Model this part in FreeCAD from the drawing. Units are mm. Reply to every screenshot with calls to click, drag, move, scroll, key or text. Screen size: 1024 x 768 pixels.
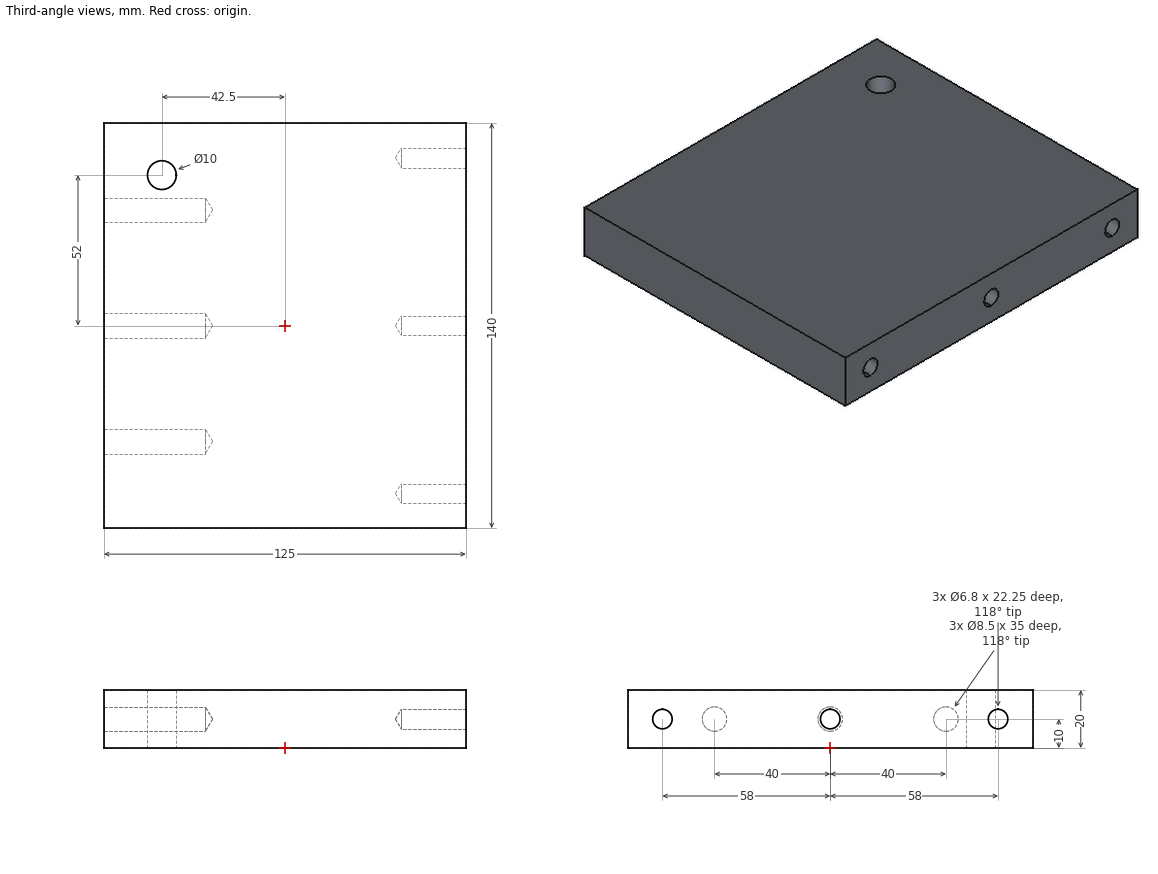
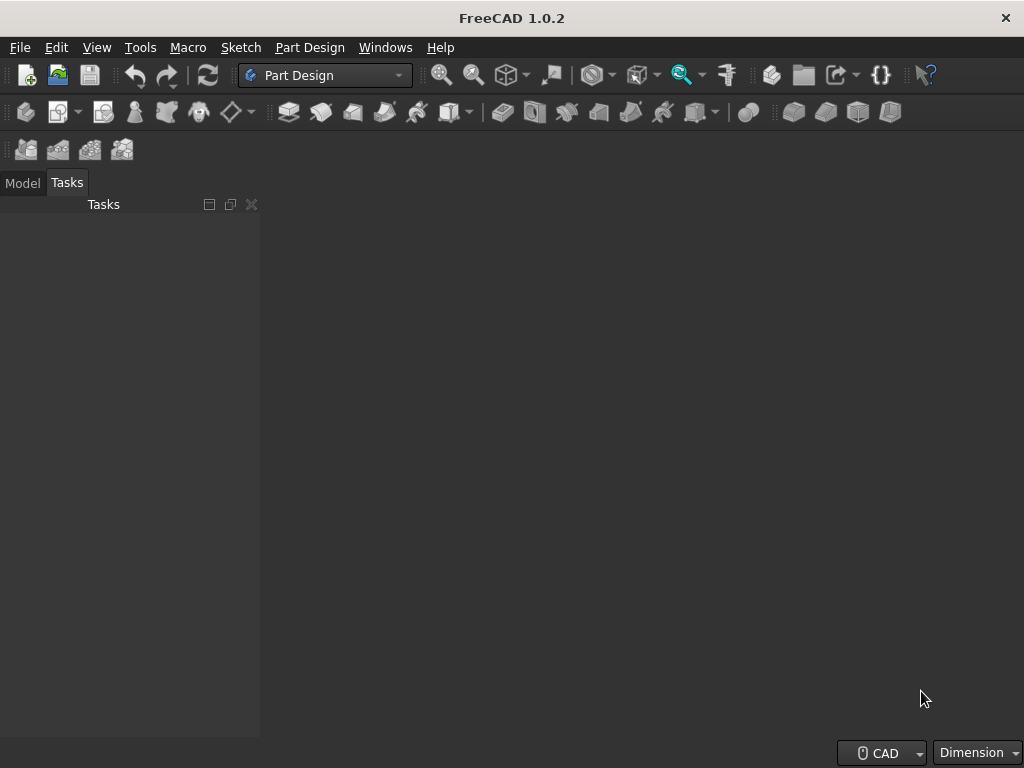
click(26, 76)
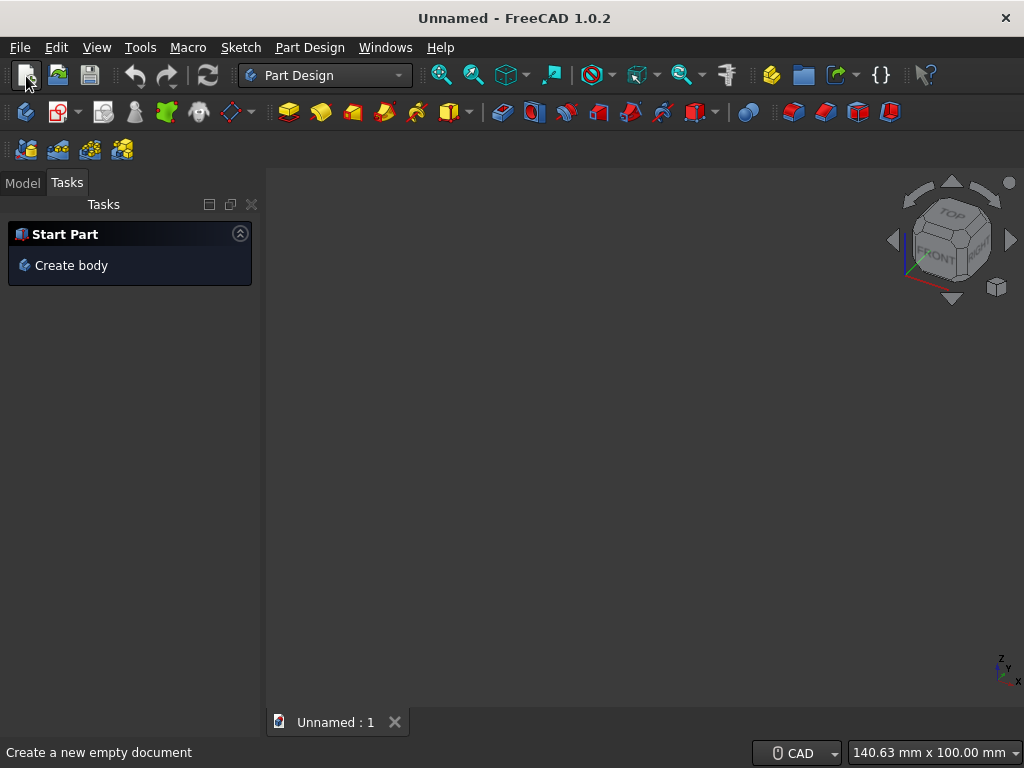
click(58, 112)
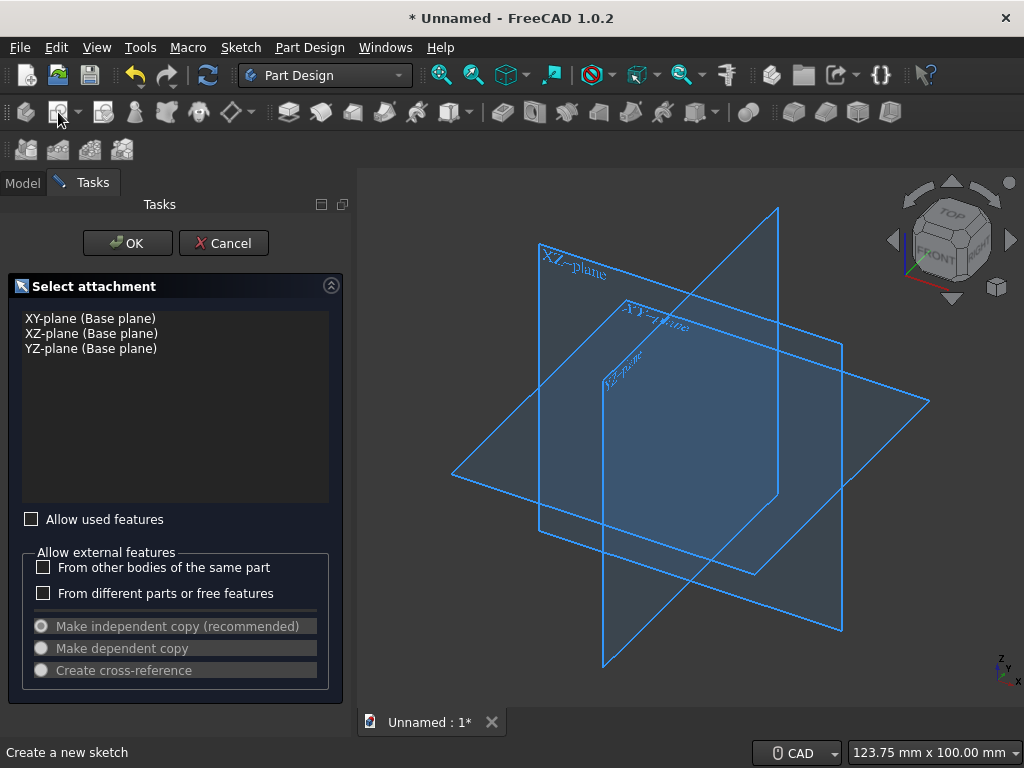
click(82, 318)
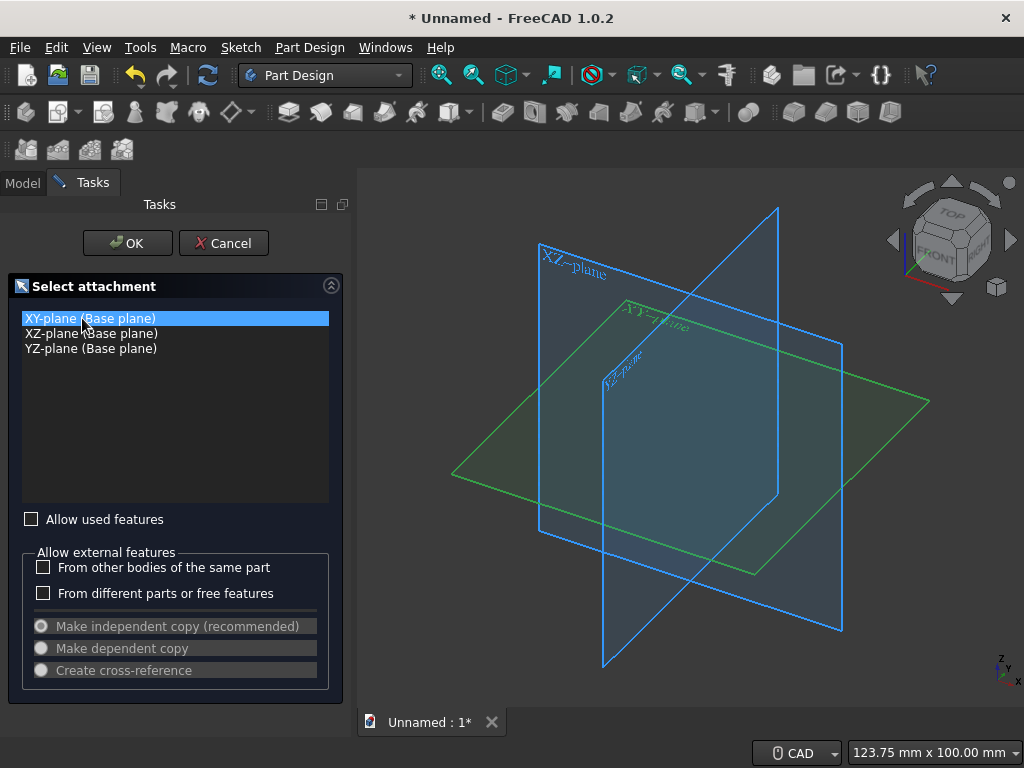
click(128, 243)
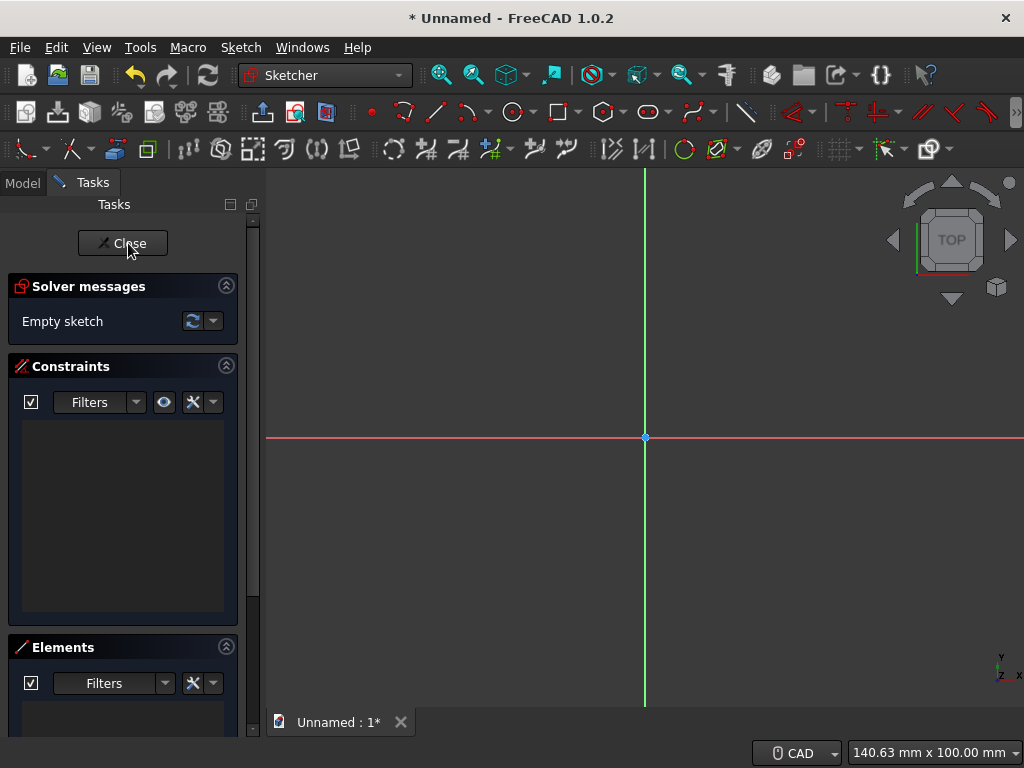
scroll(521, 438, down, 4)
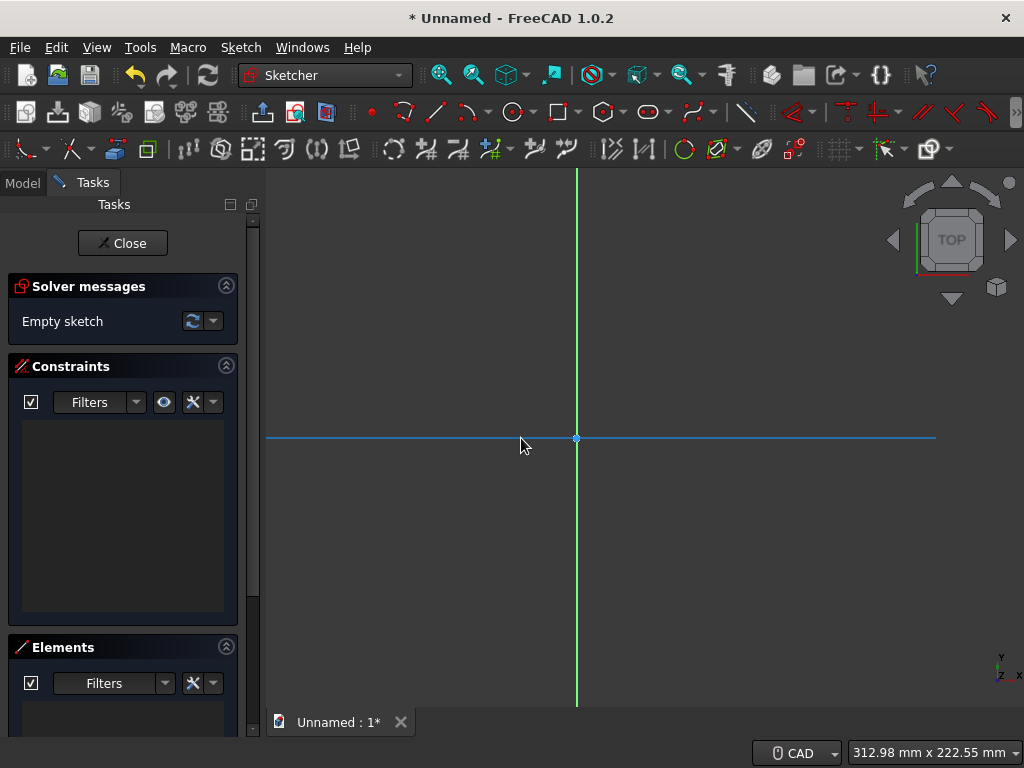
click(580, 112)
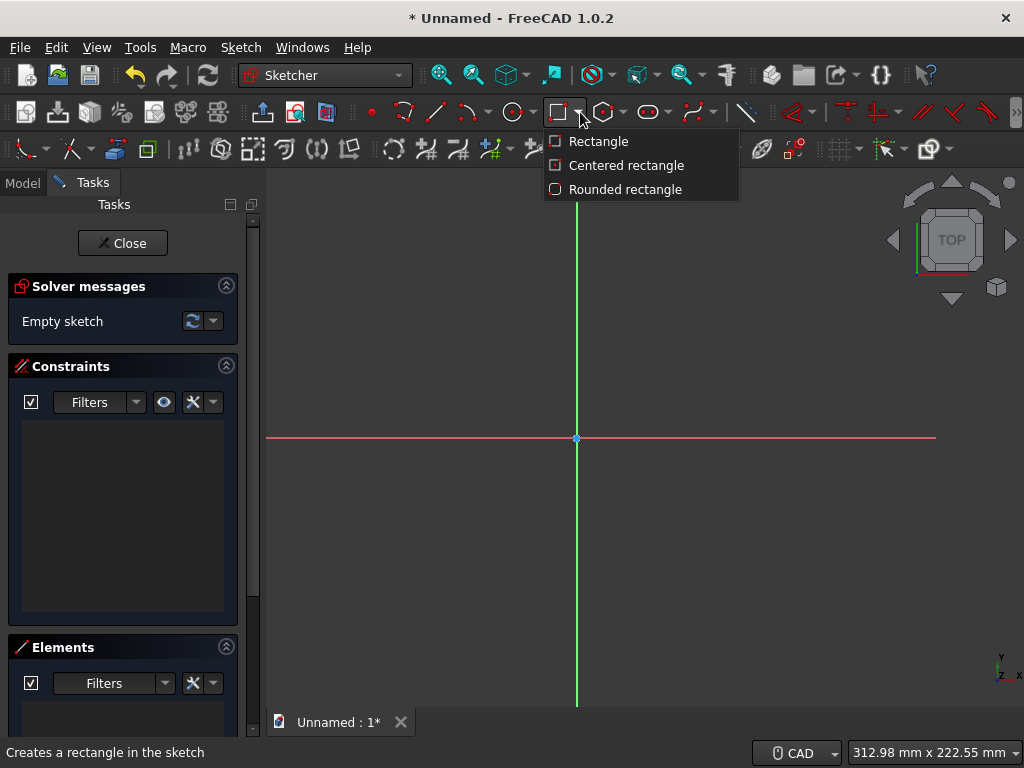
click(642, 165)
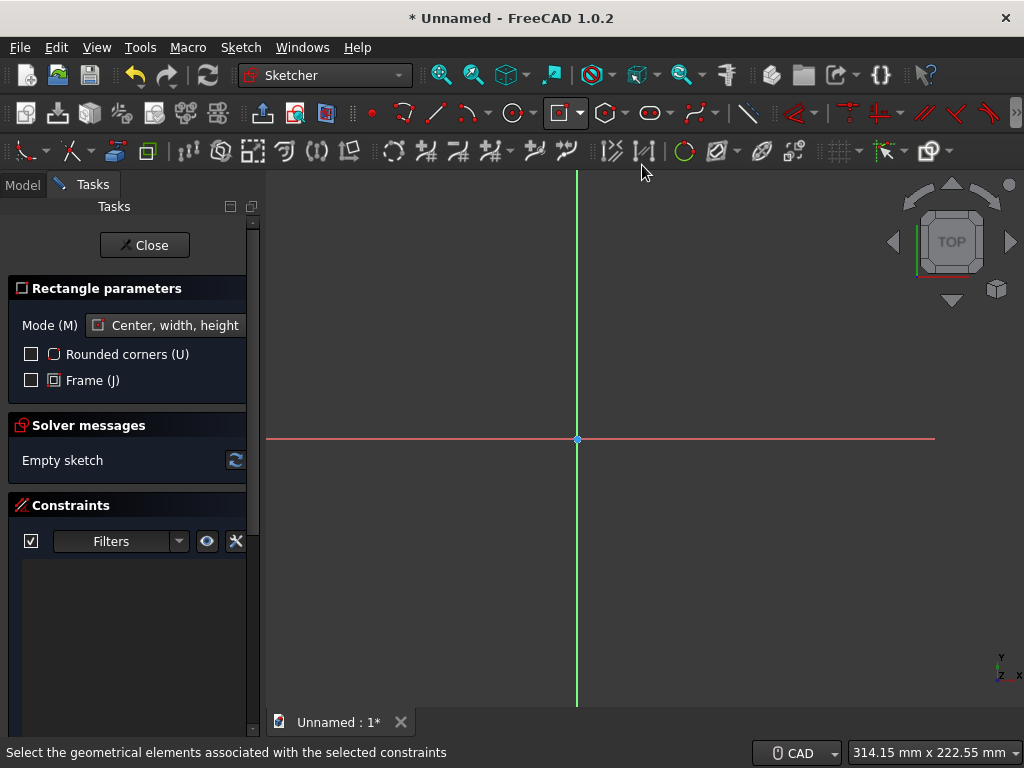
click(577, 439)
click(728, 270)
key(Escape)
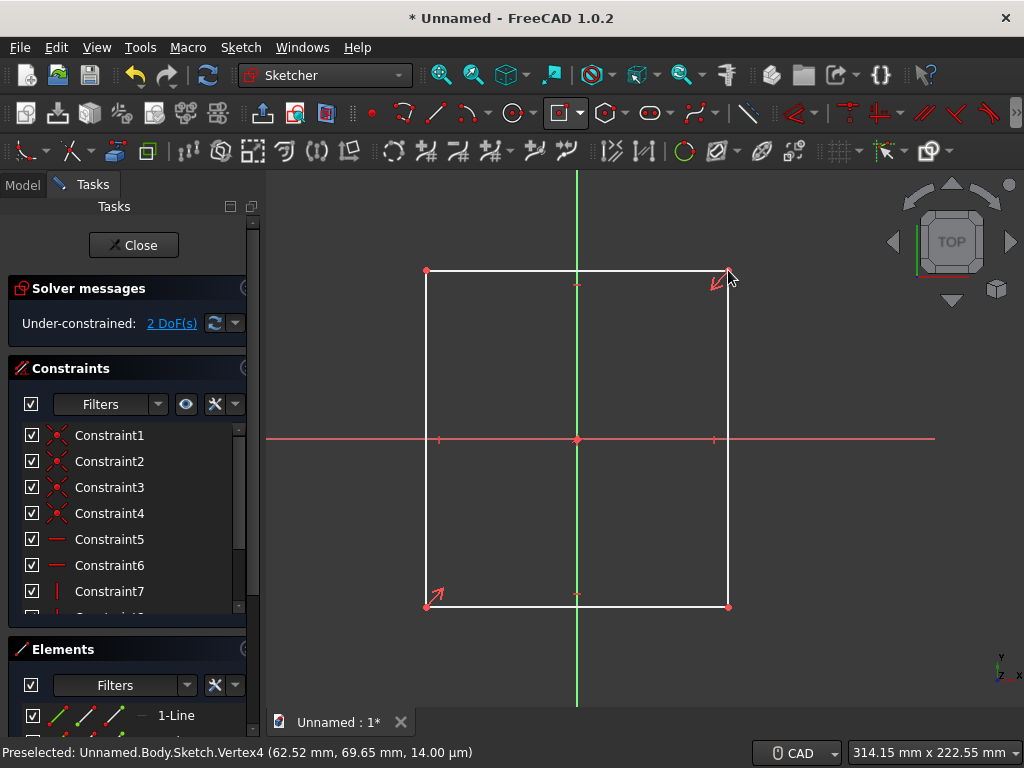
click(794, 114)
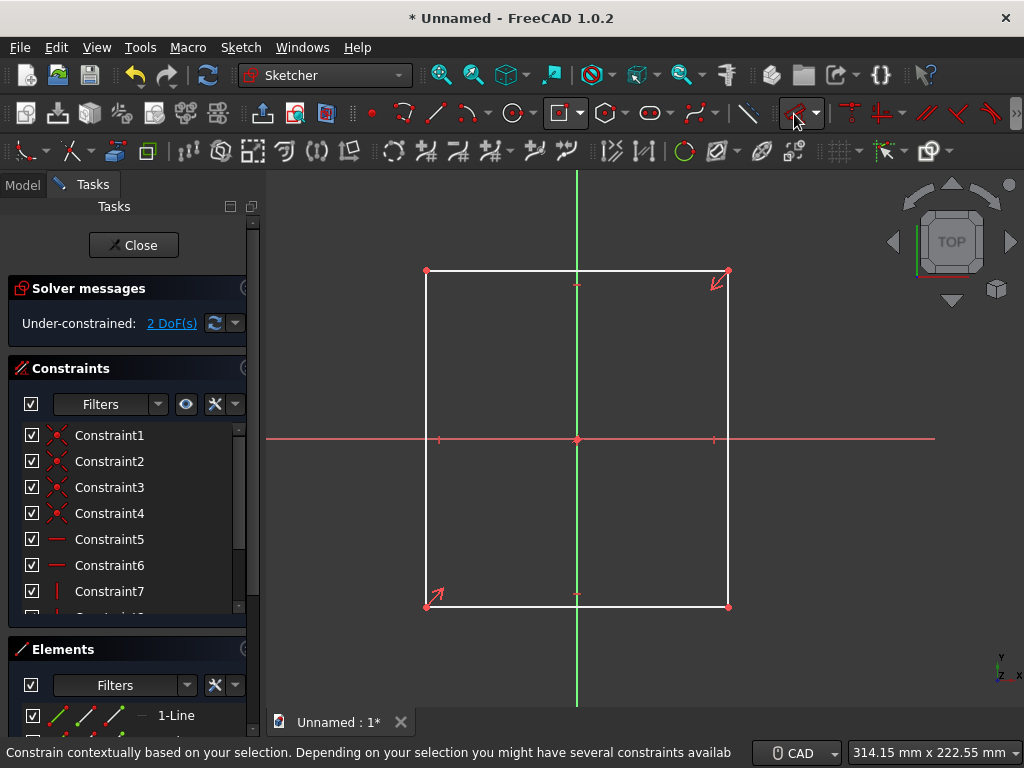
click(517, 607)
click(508, 641)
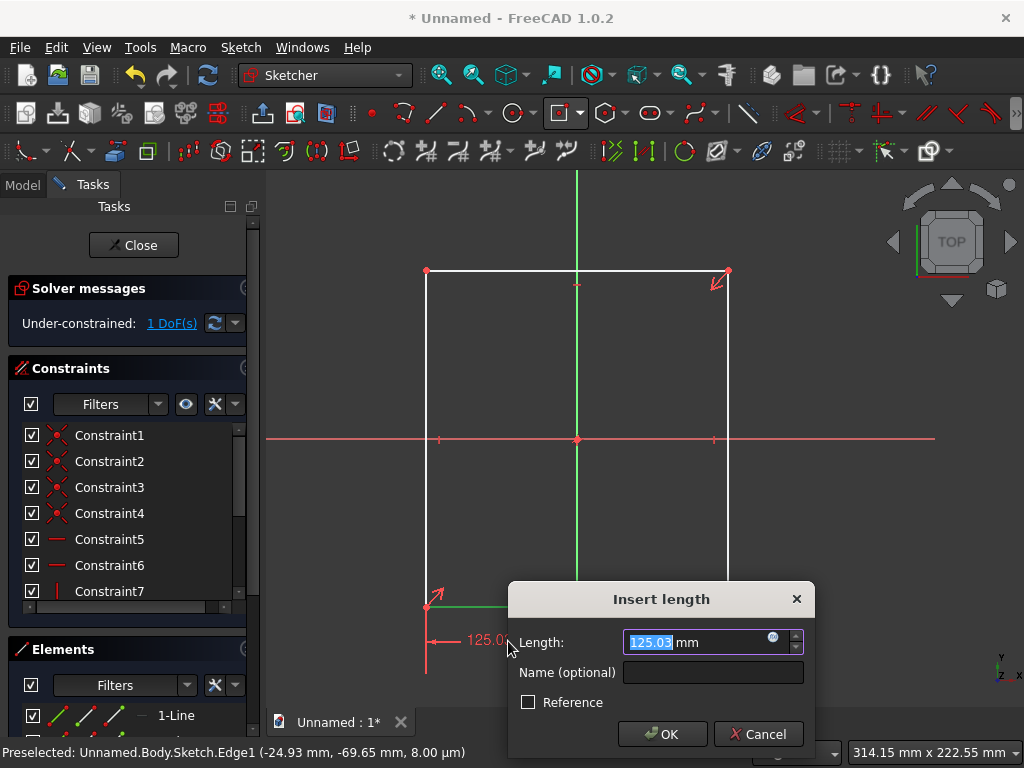
text(125)
key(Return)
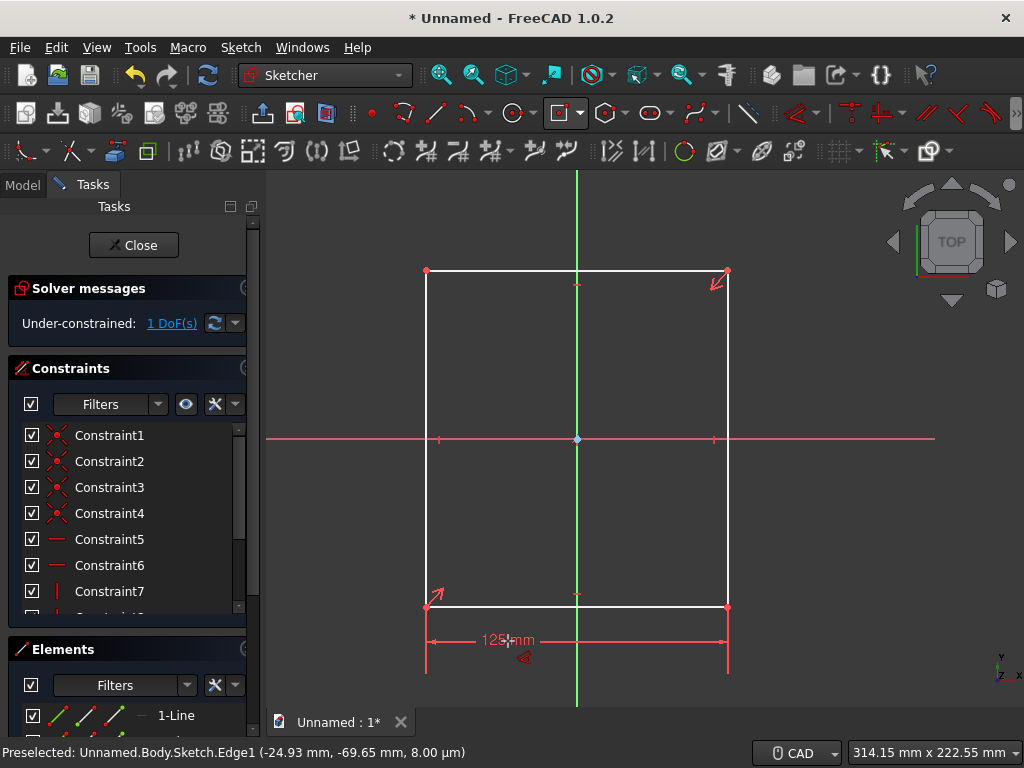
click(728, 506)
click(762, 362)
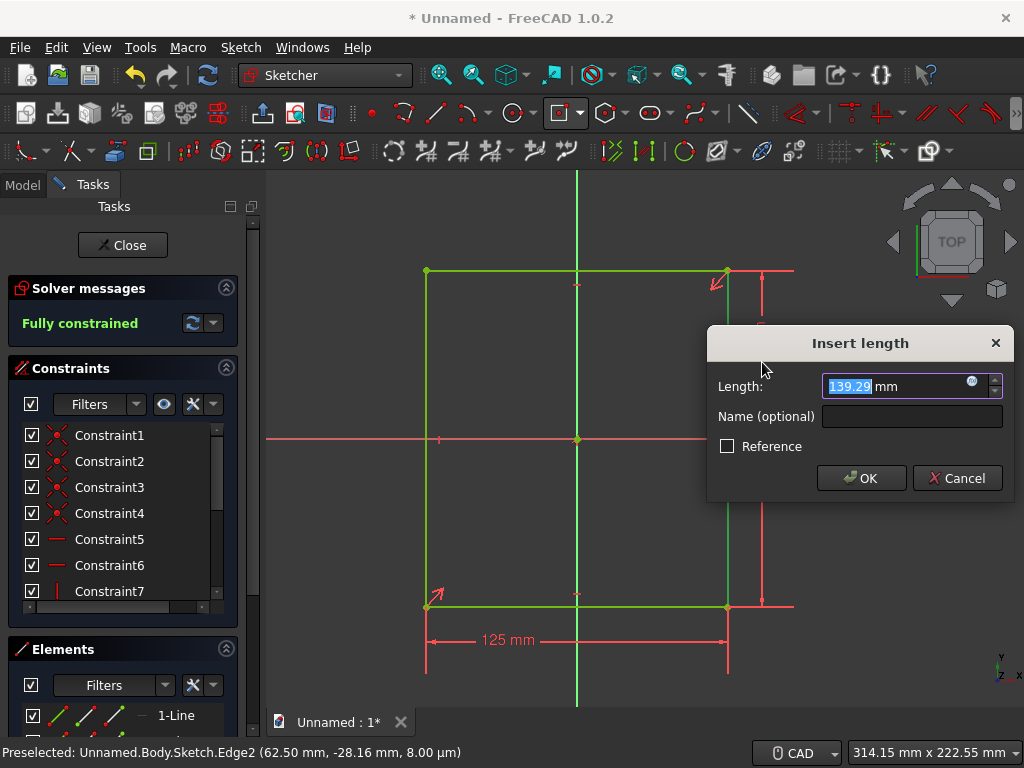
text(140)
key(Return)
key(Escape)